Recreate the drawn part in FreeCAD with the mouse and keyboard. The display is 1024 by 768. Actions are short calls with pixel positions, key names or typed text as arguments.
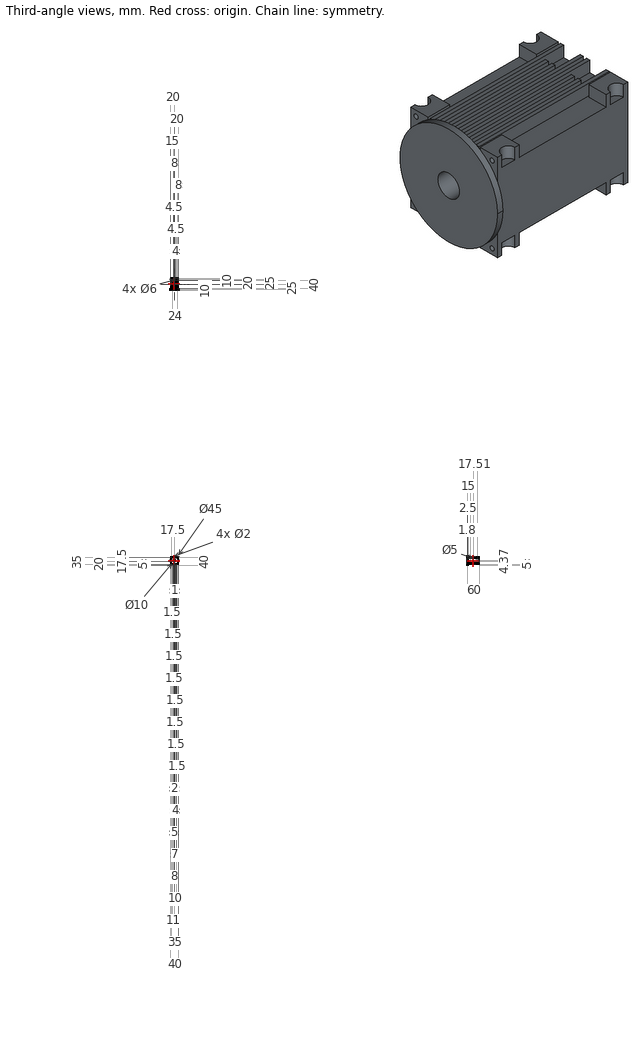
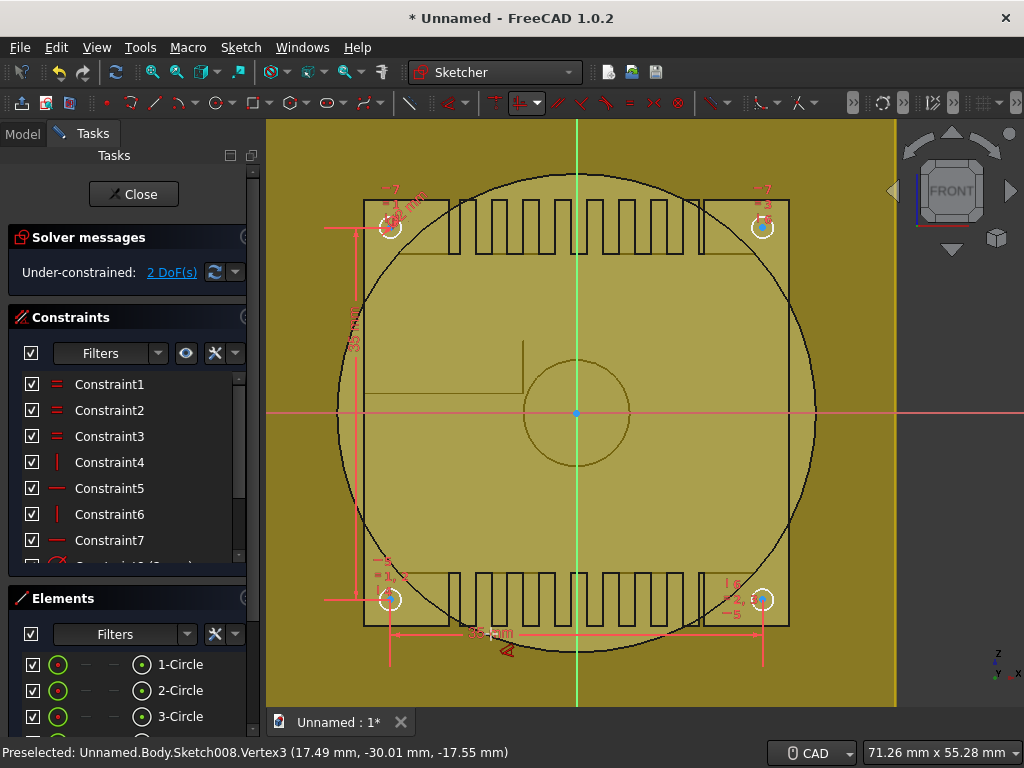
click(390, 228)
click(483, 194)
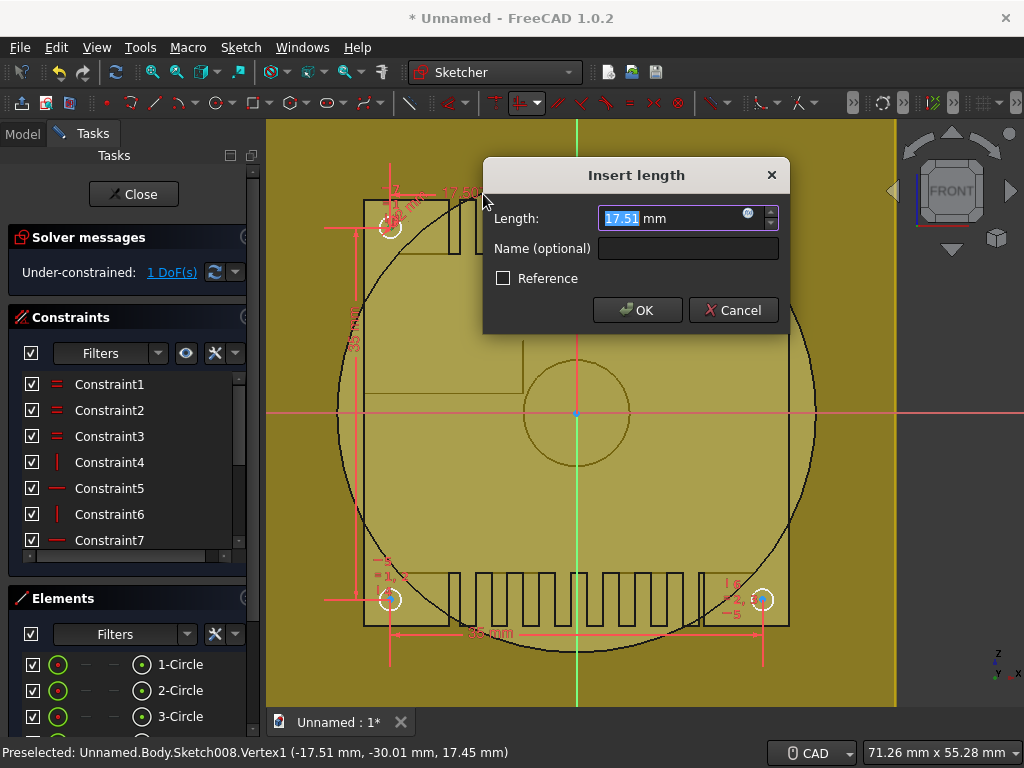
text(17.5)
key(Return)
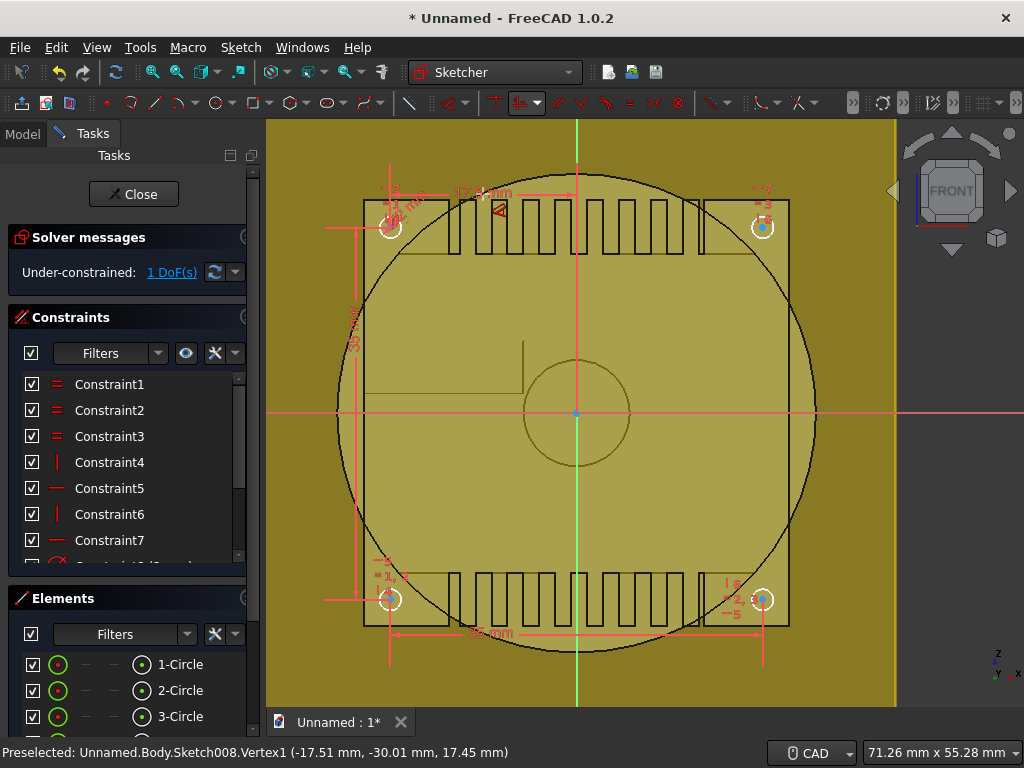
click(390, 228)
click(356, 278)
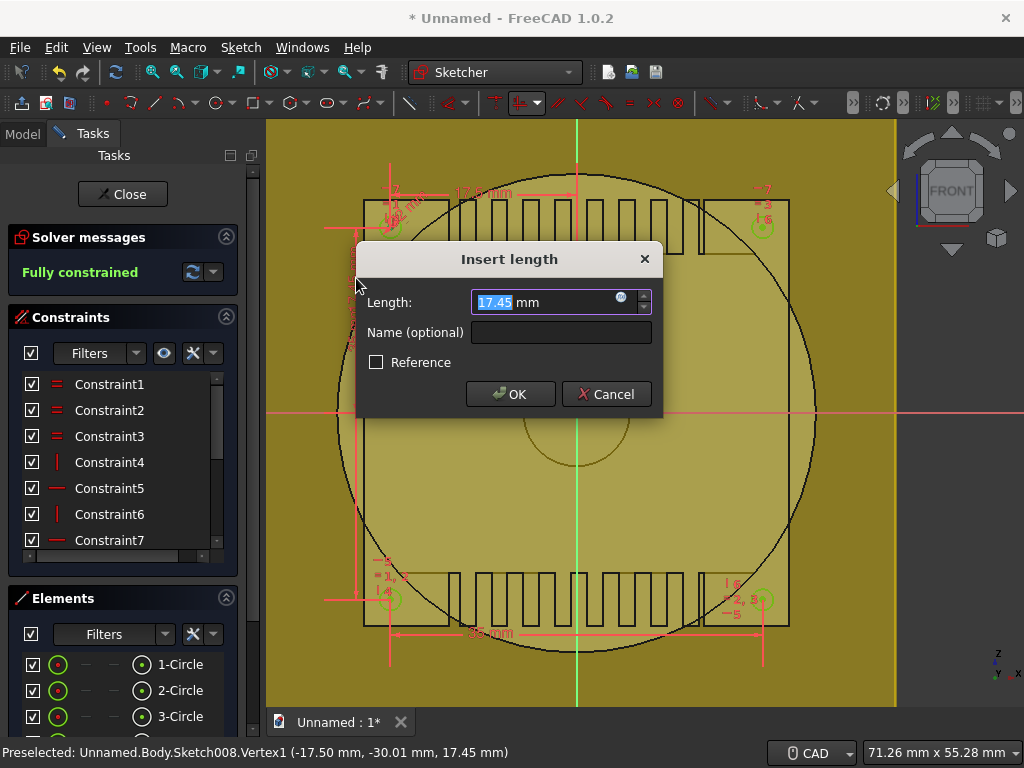
text(17.5)
key(Return)
key(Escape)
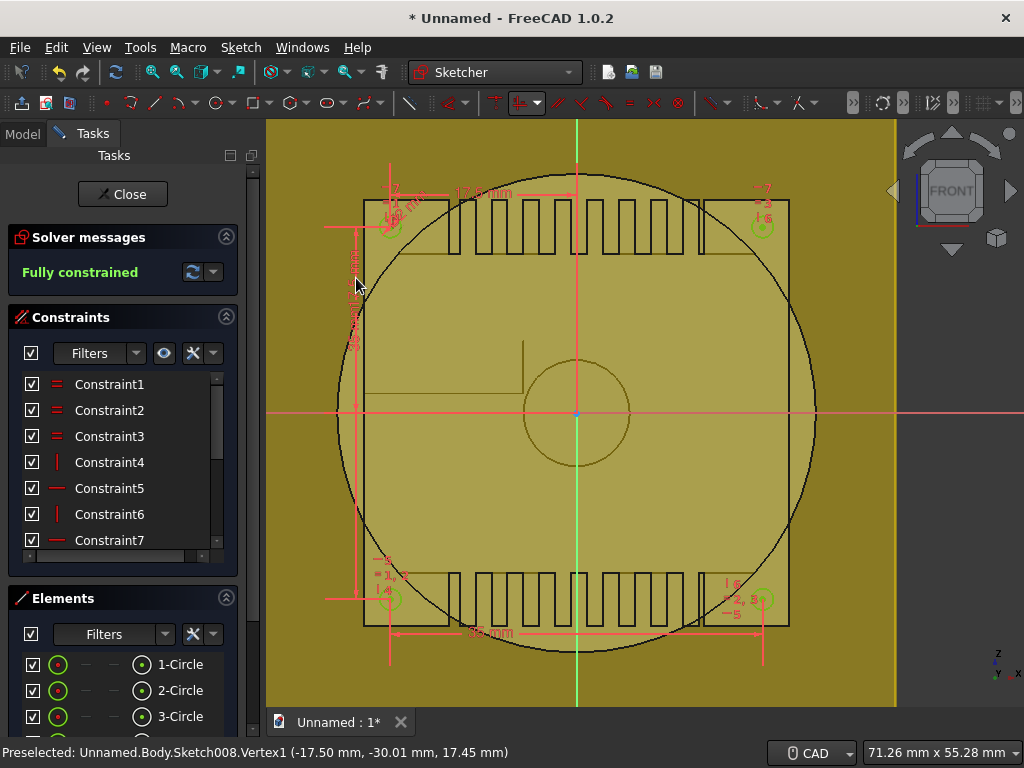
click(123, 194)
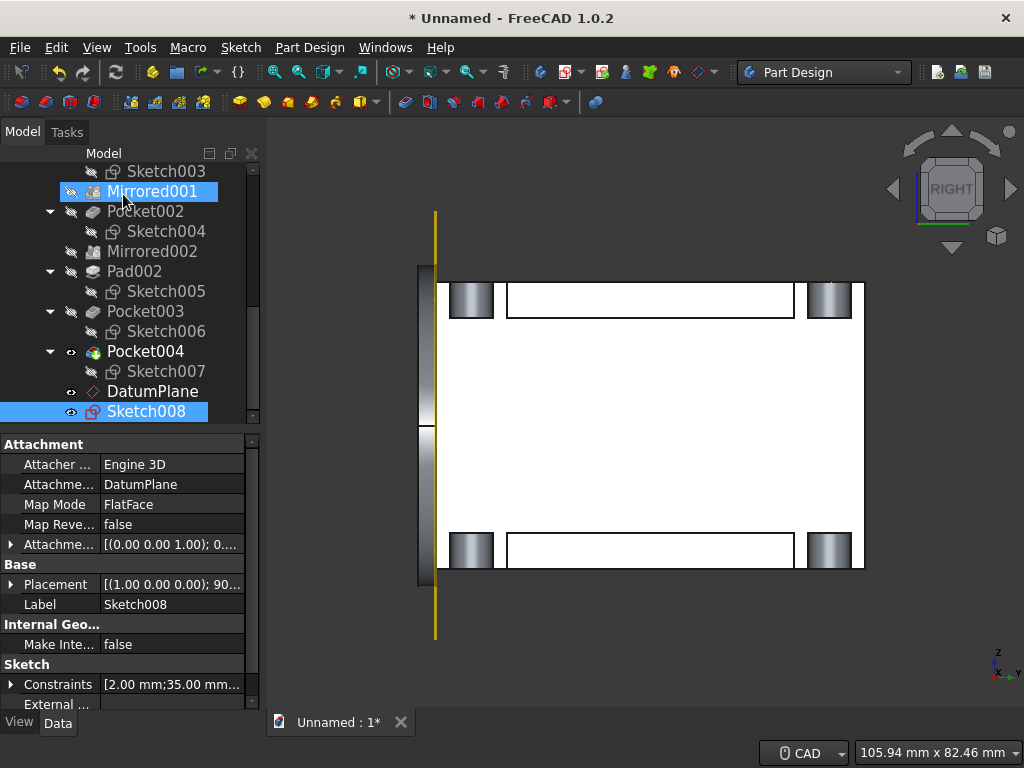
click(406, 102)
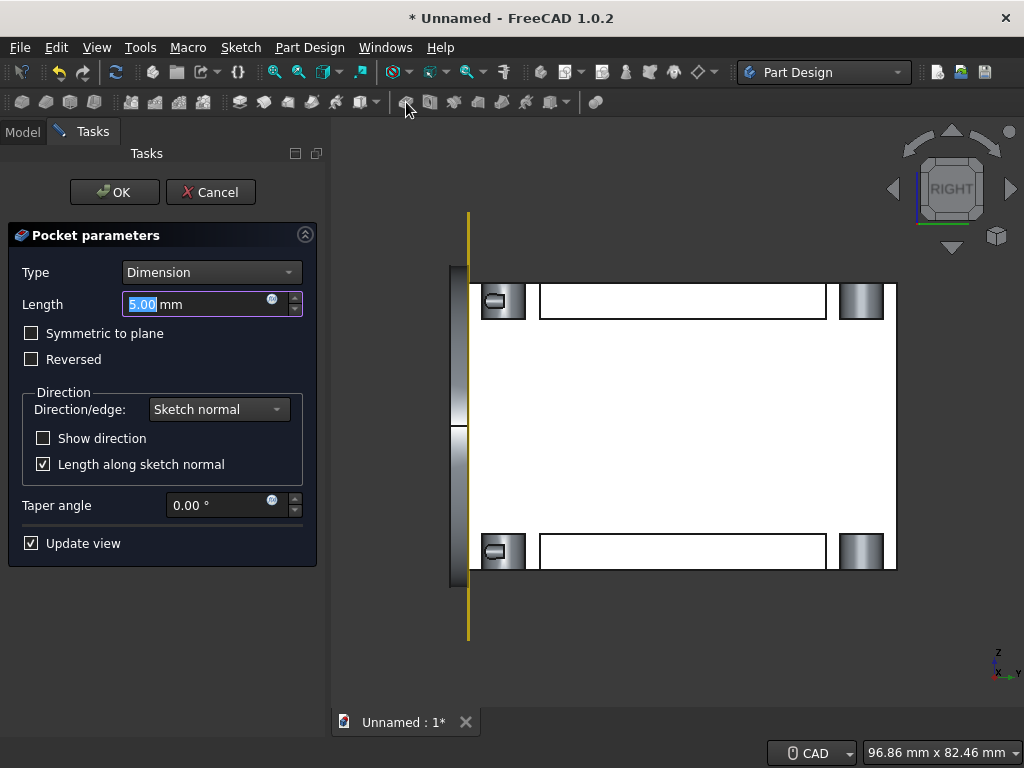
text(1.8)
key(Tab)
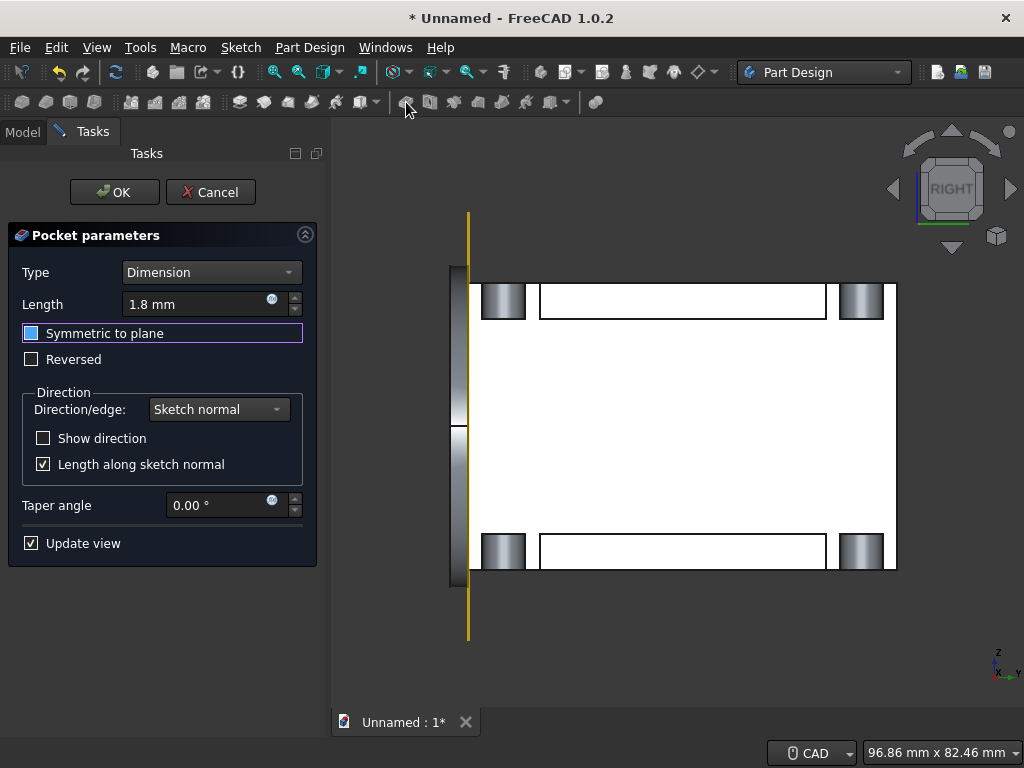
click(115, 192)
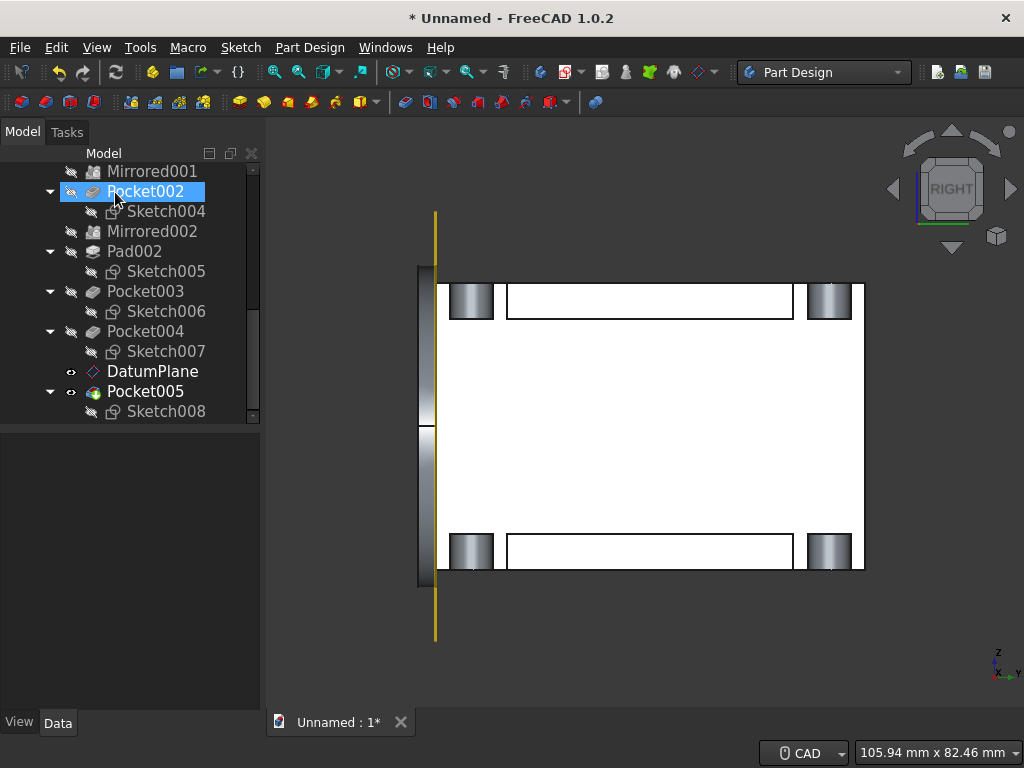
click(116, 372)
key(space)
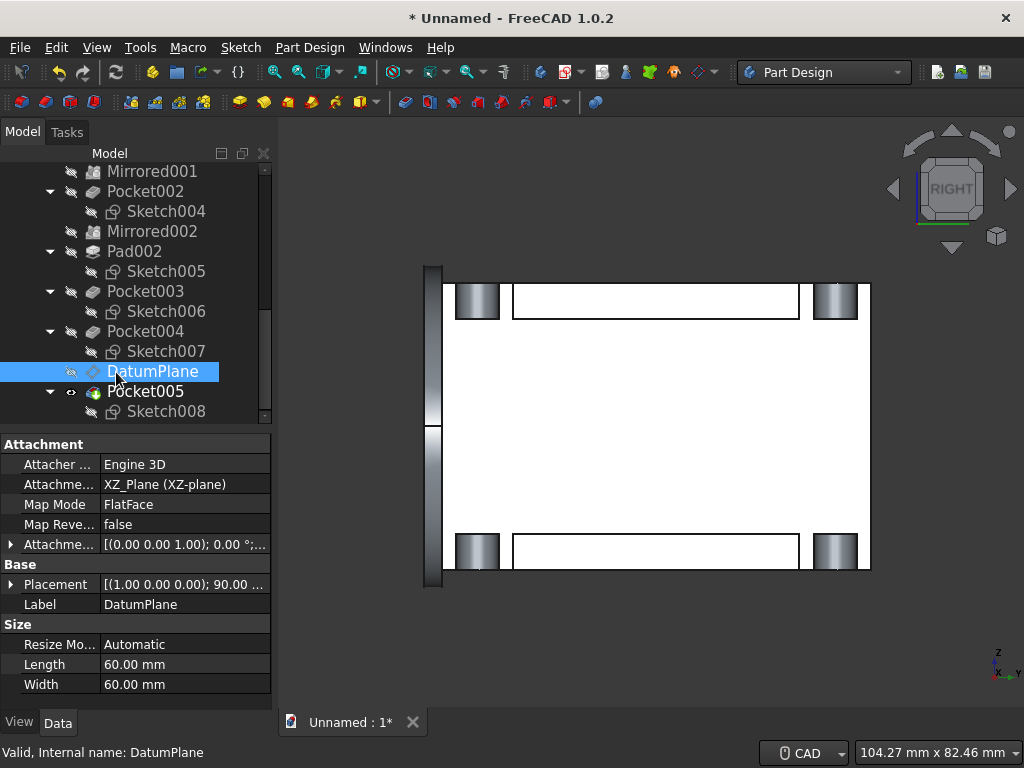
key(0)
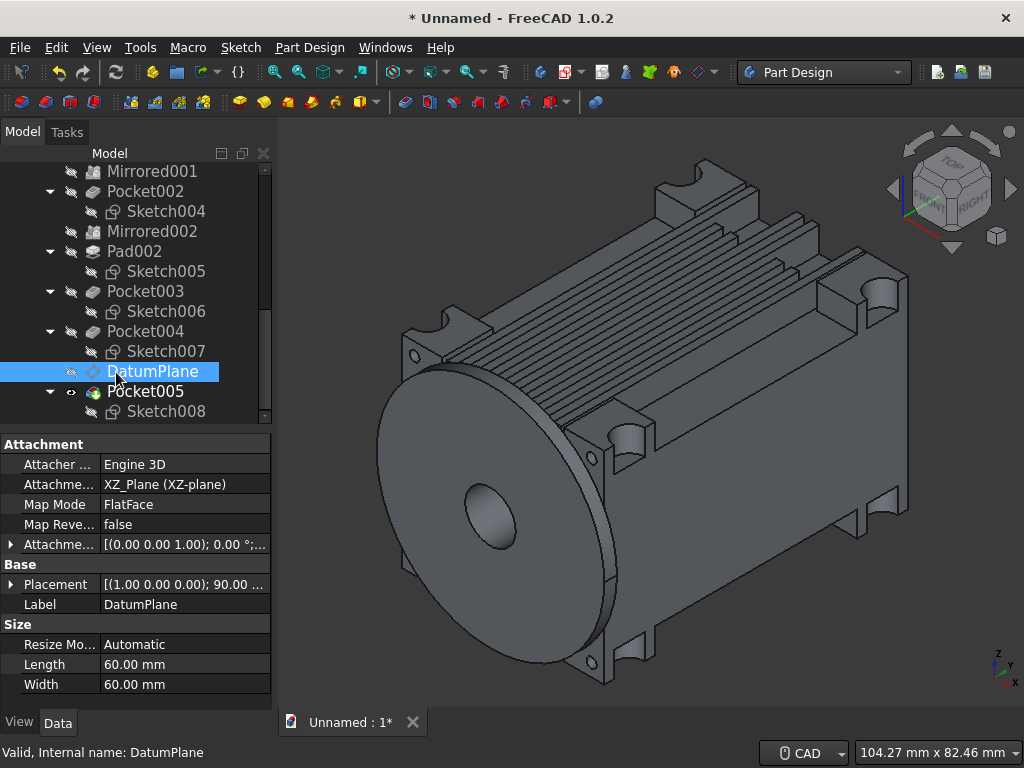
key(v)
key(f)